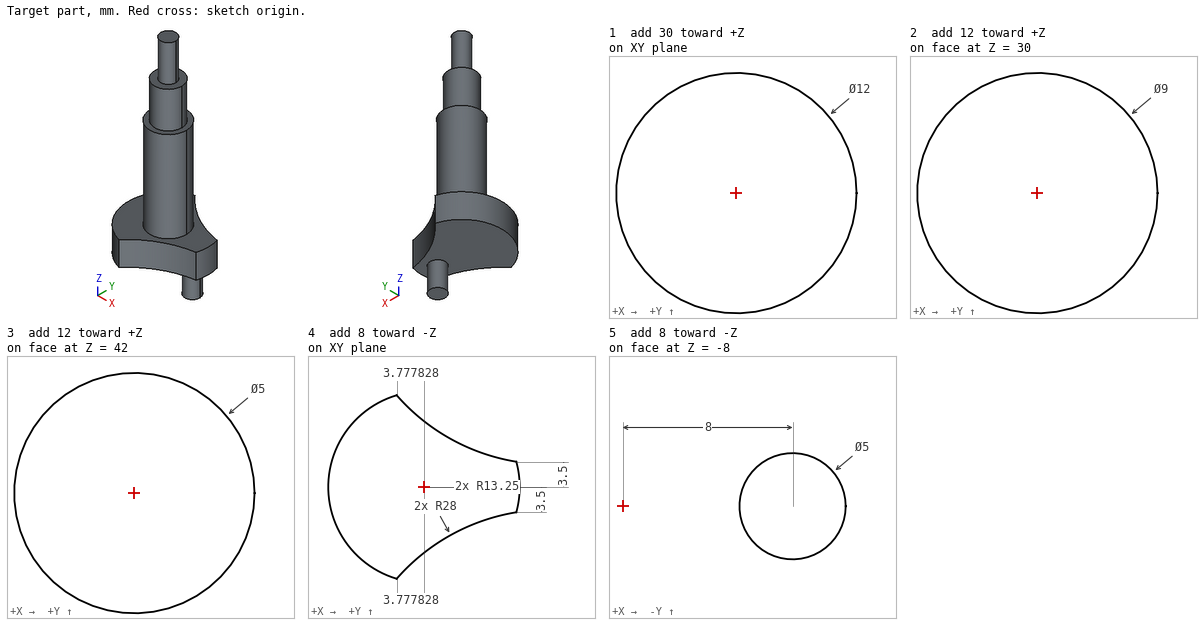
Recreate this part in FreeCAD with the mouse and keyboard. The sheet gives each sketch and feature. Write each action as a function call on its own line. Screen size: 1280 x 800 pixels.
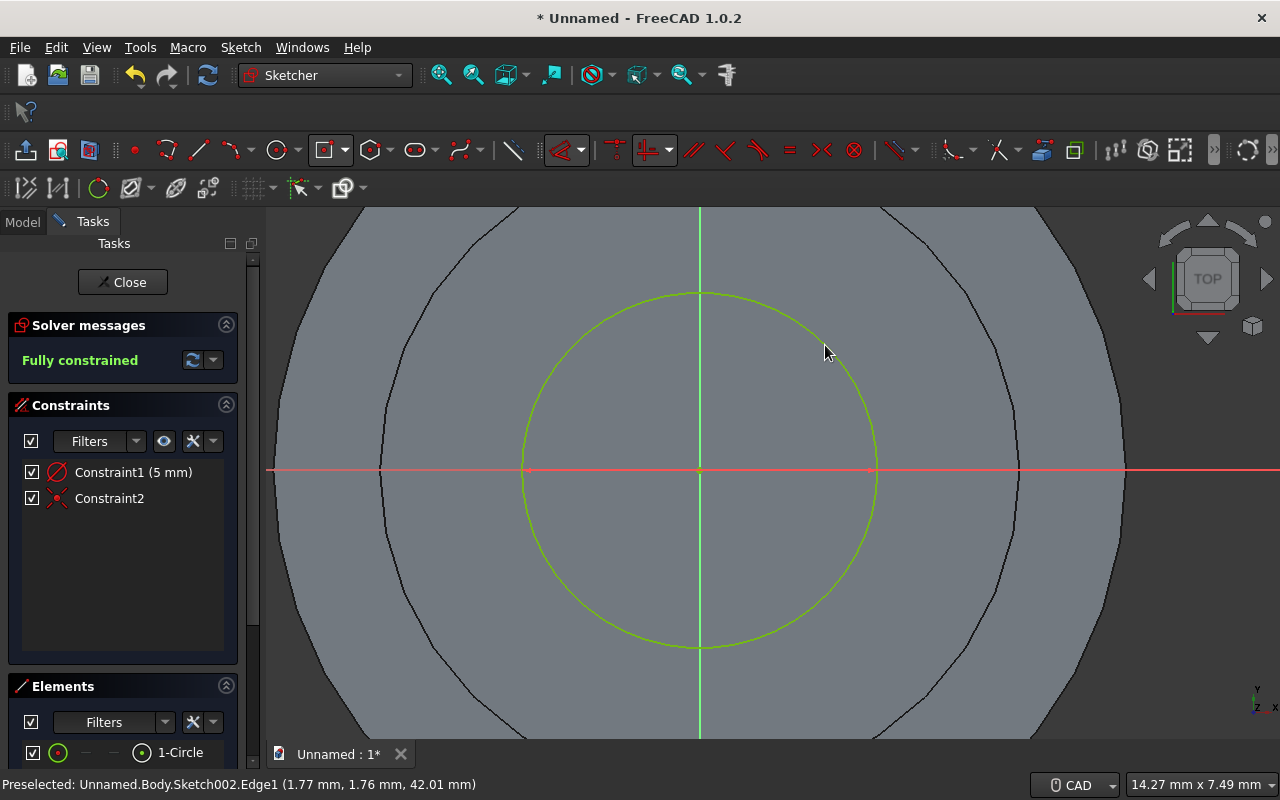
click(123, 282)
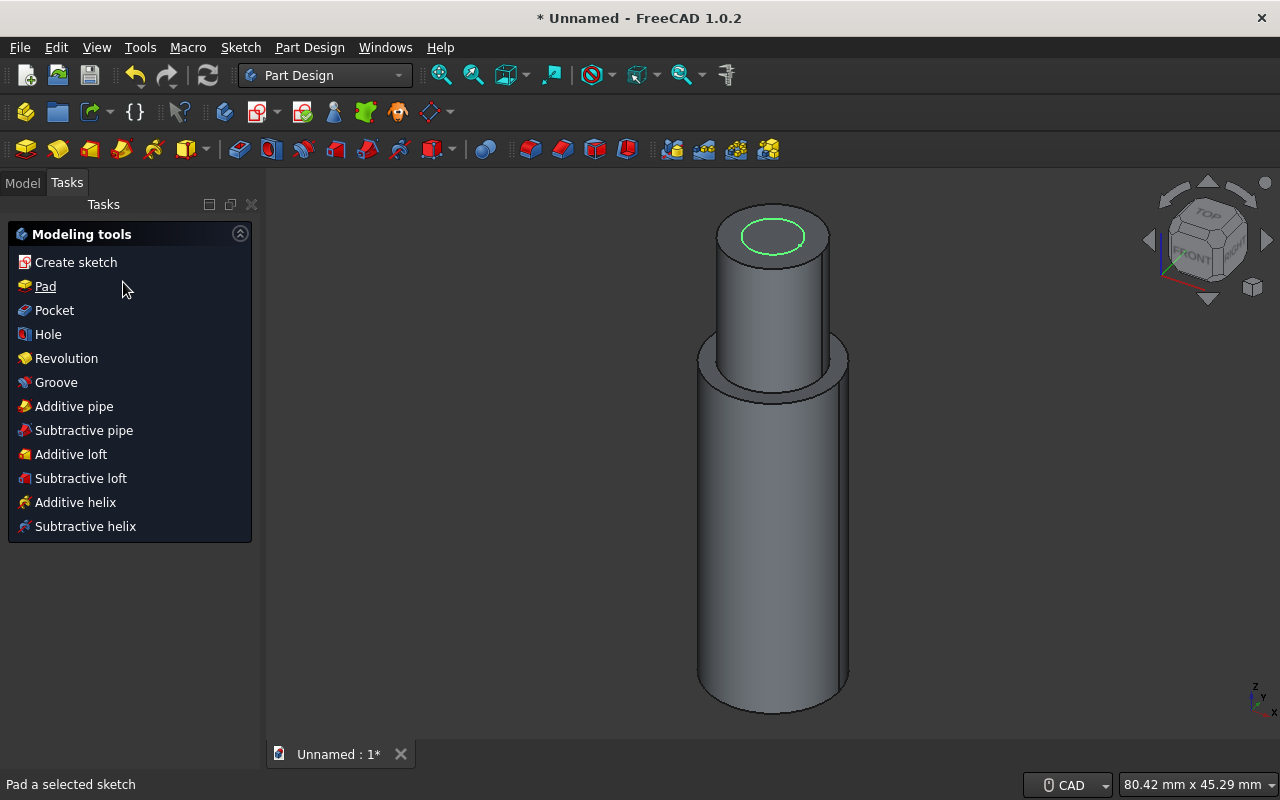
click(26, 150)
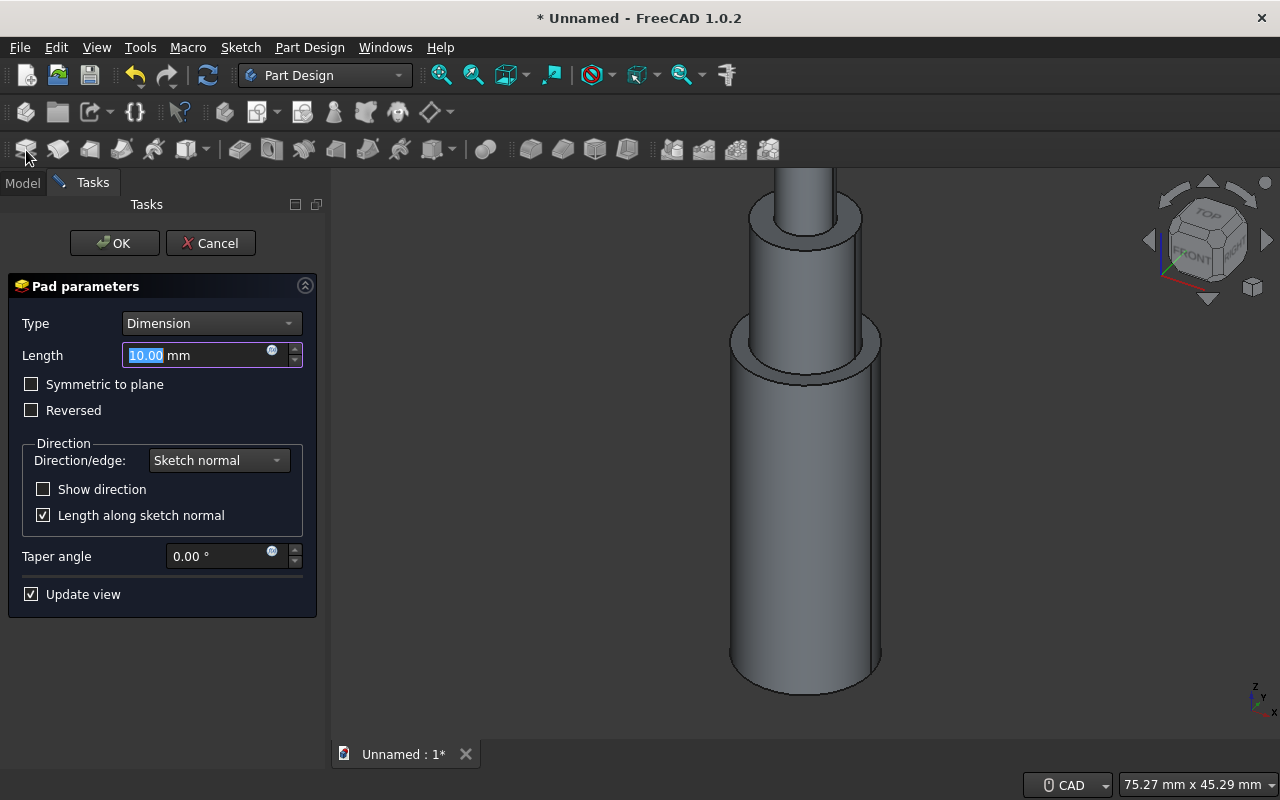
text(12)
key(Tab)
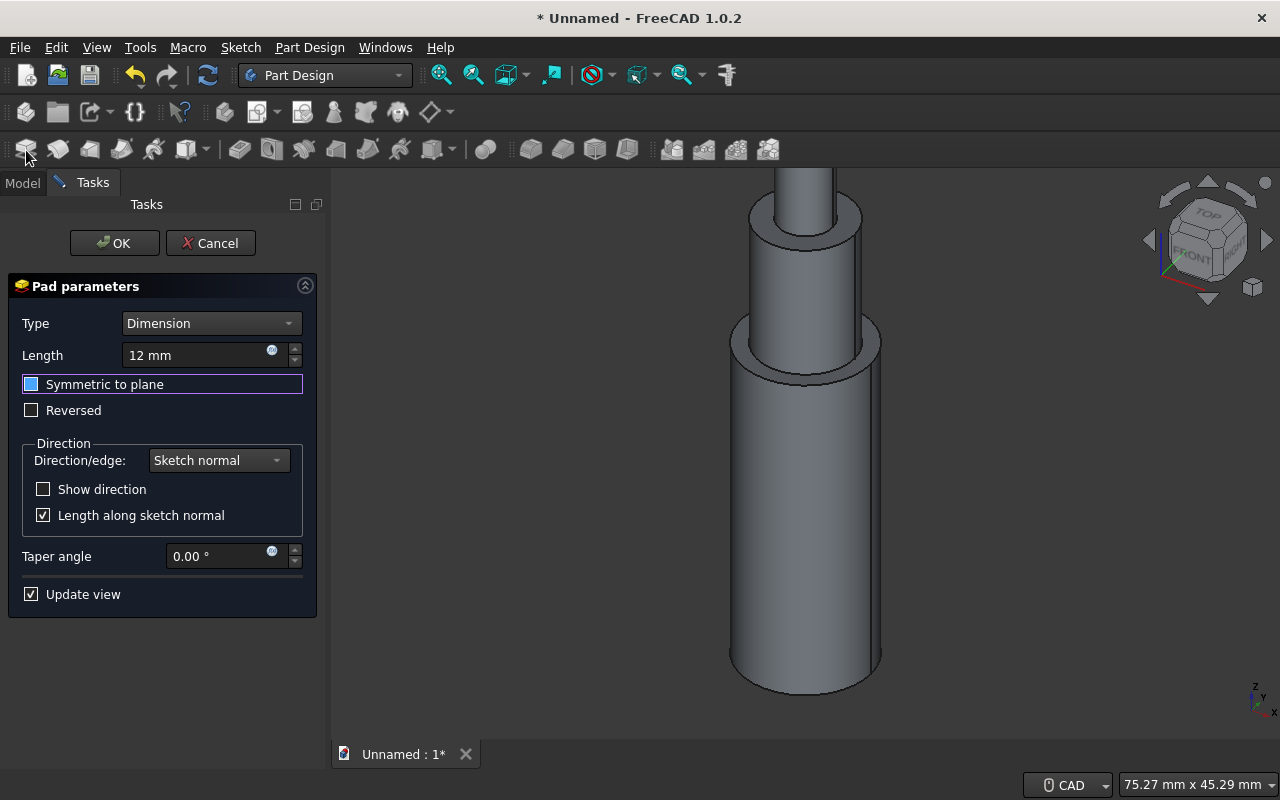
click(115, 243)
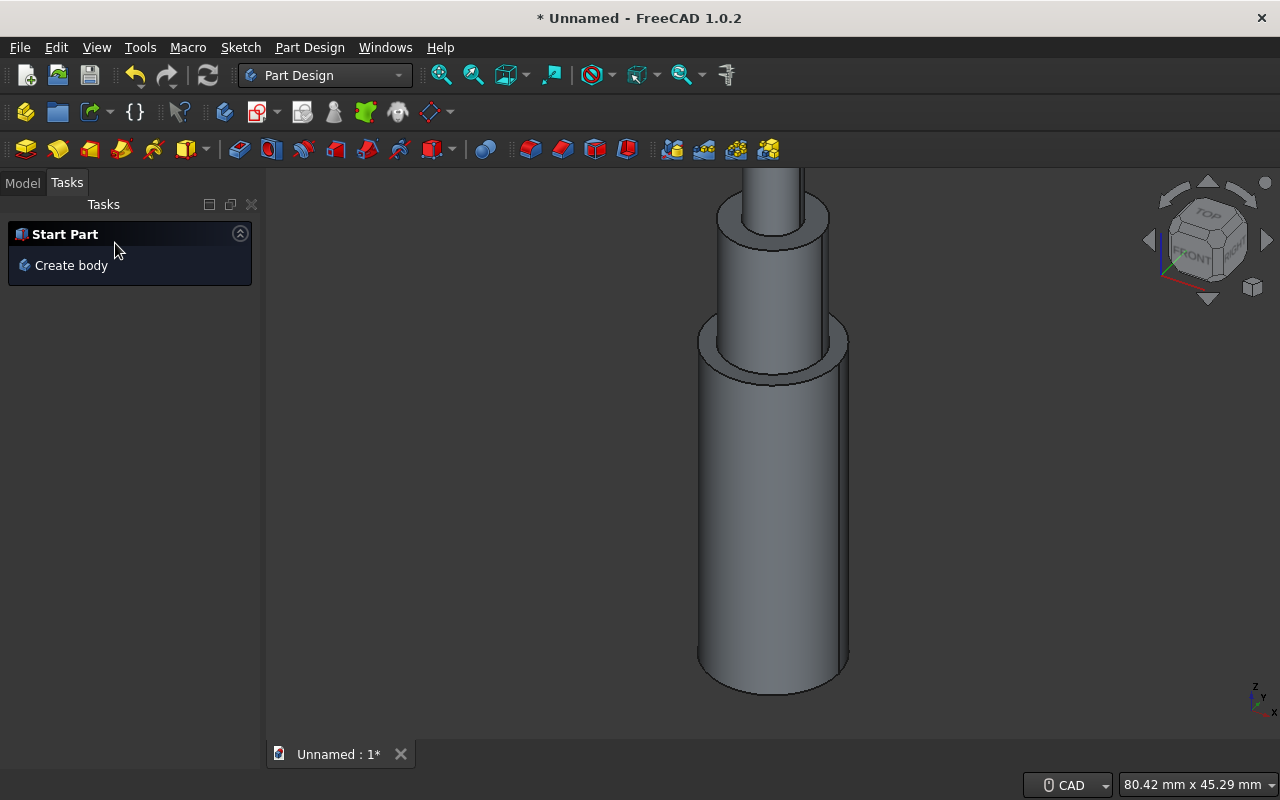
click(442, 76)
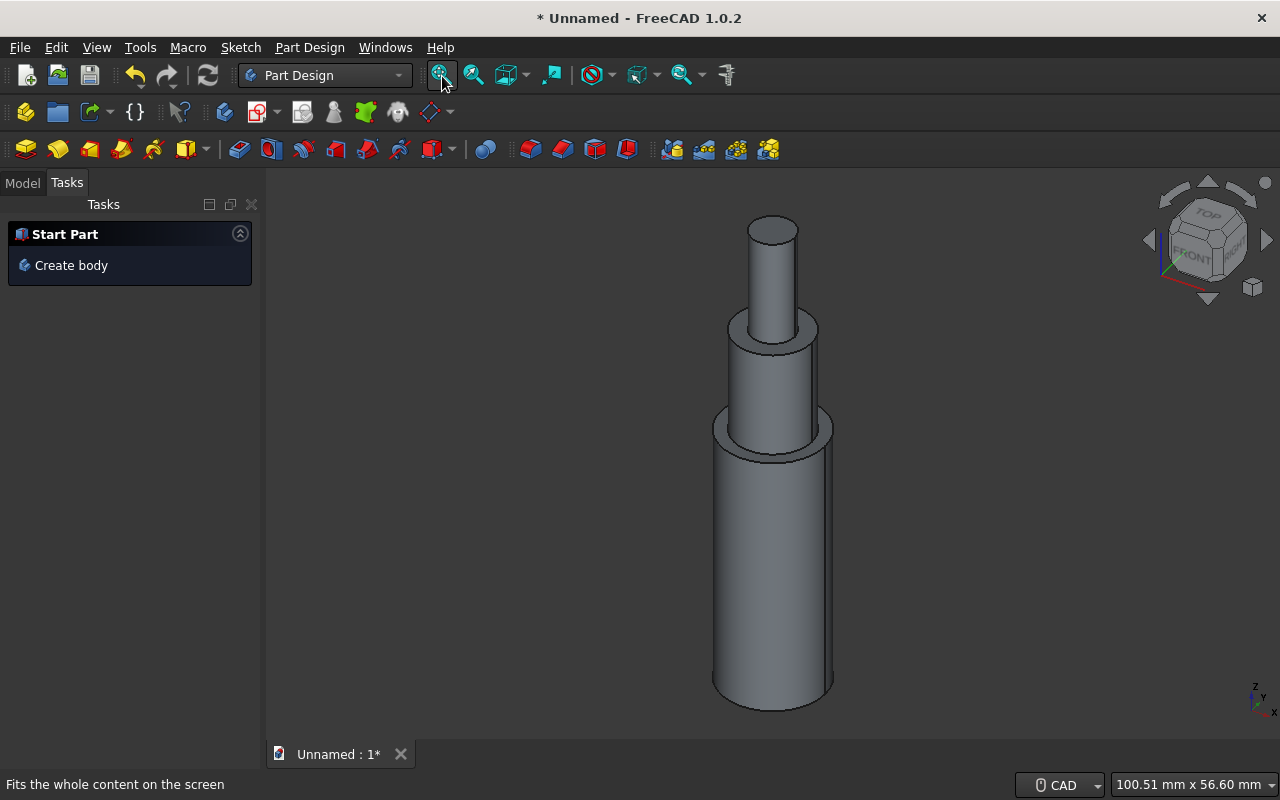
click(258, 112)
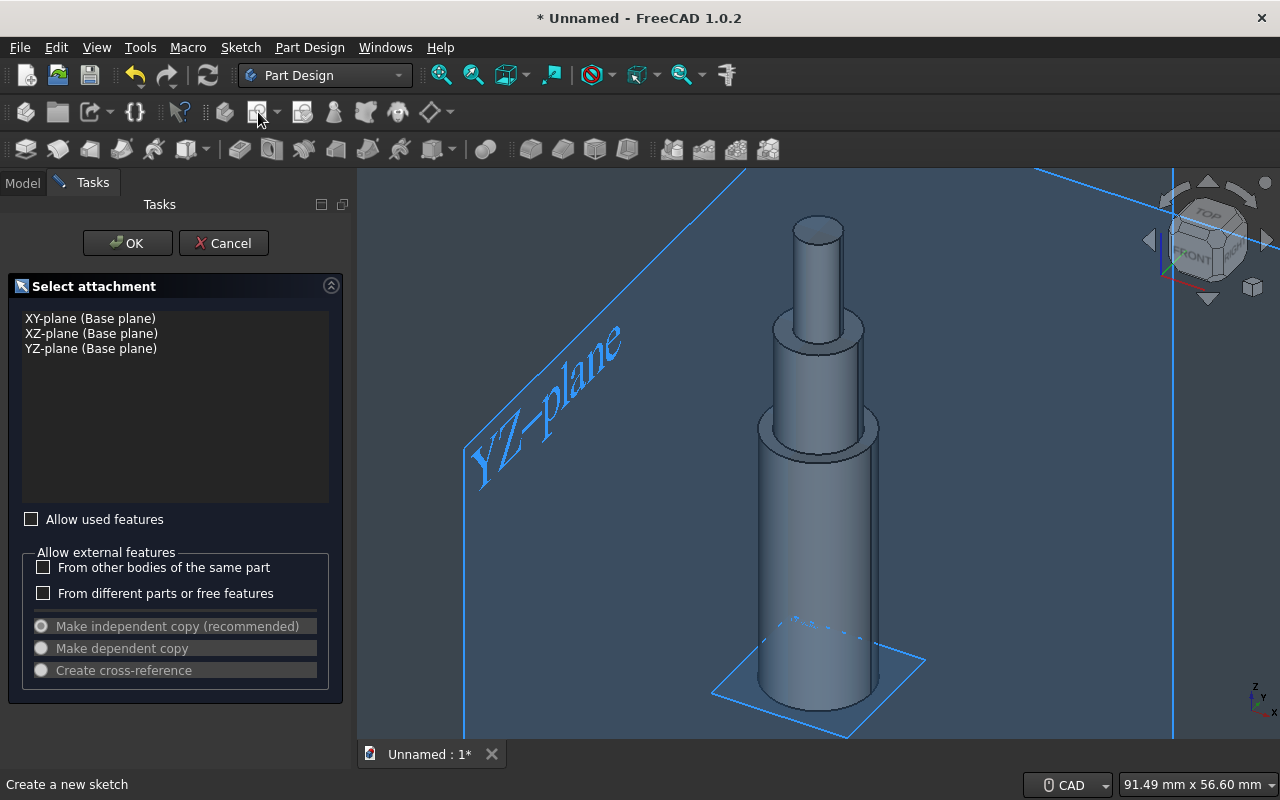
click(82, 318)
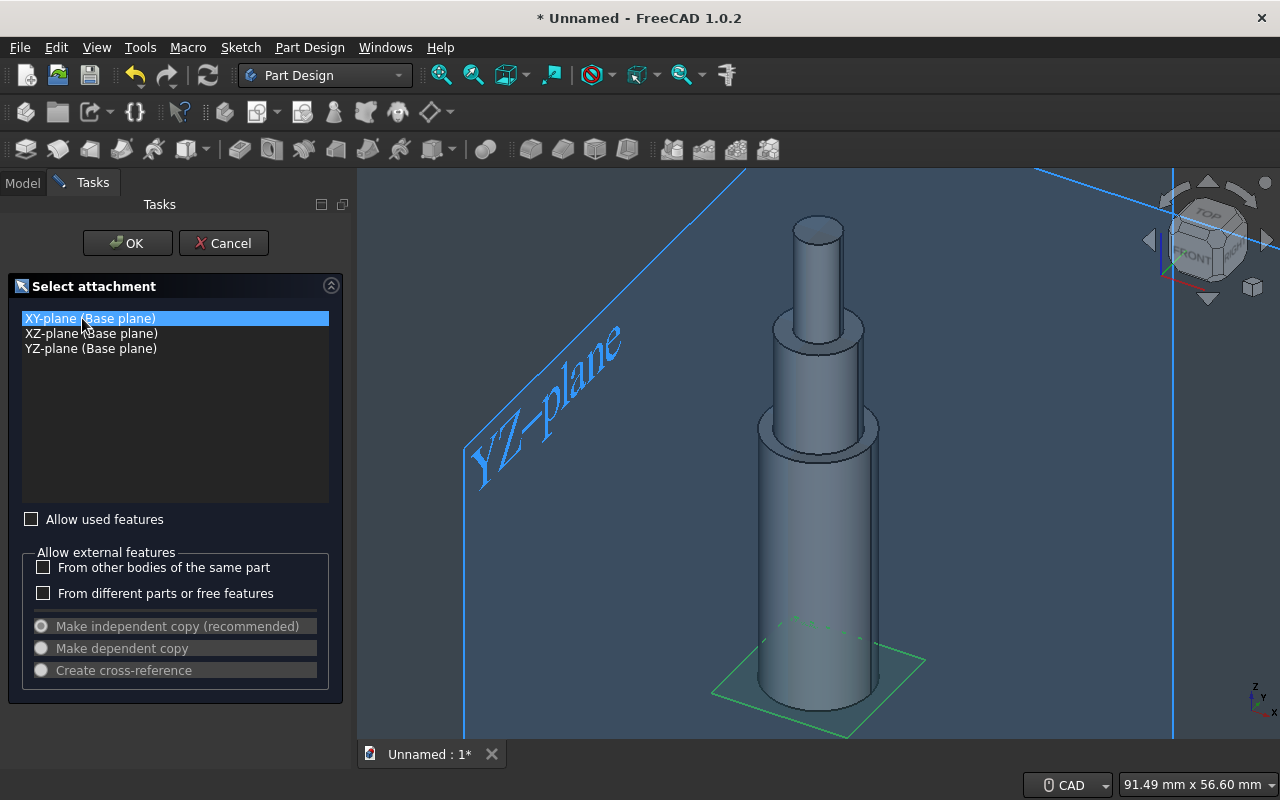
click(128, 243)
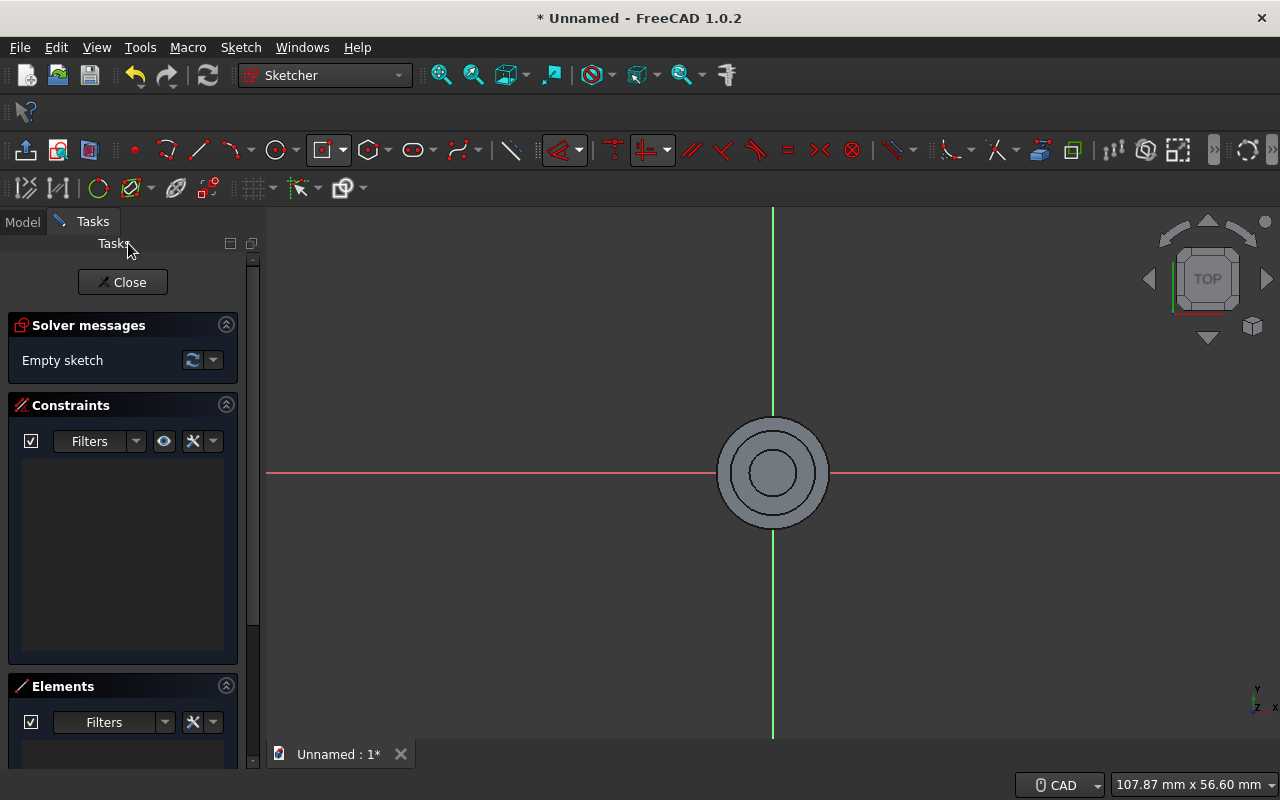
click(90, 150)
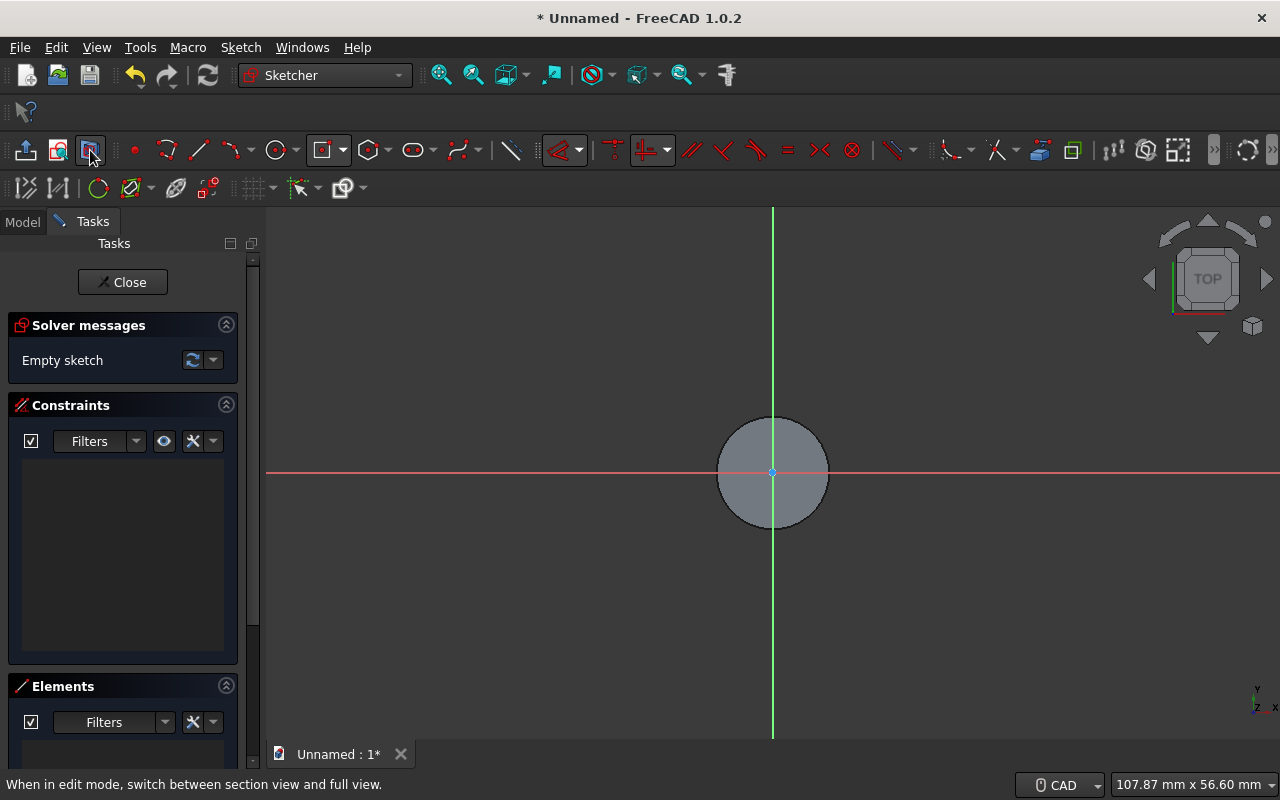
scroll(912, 473, up, 2)